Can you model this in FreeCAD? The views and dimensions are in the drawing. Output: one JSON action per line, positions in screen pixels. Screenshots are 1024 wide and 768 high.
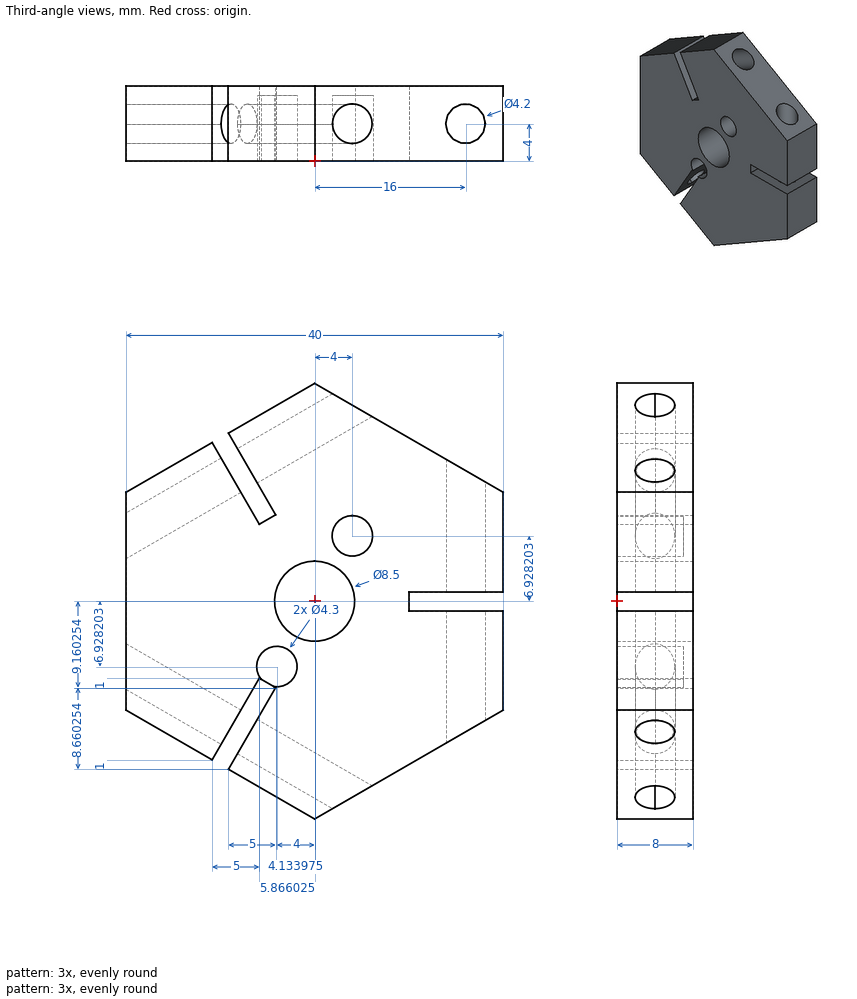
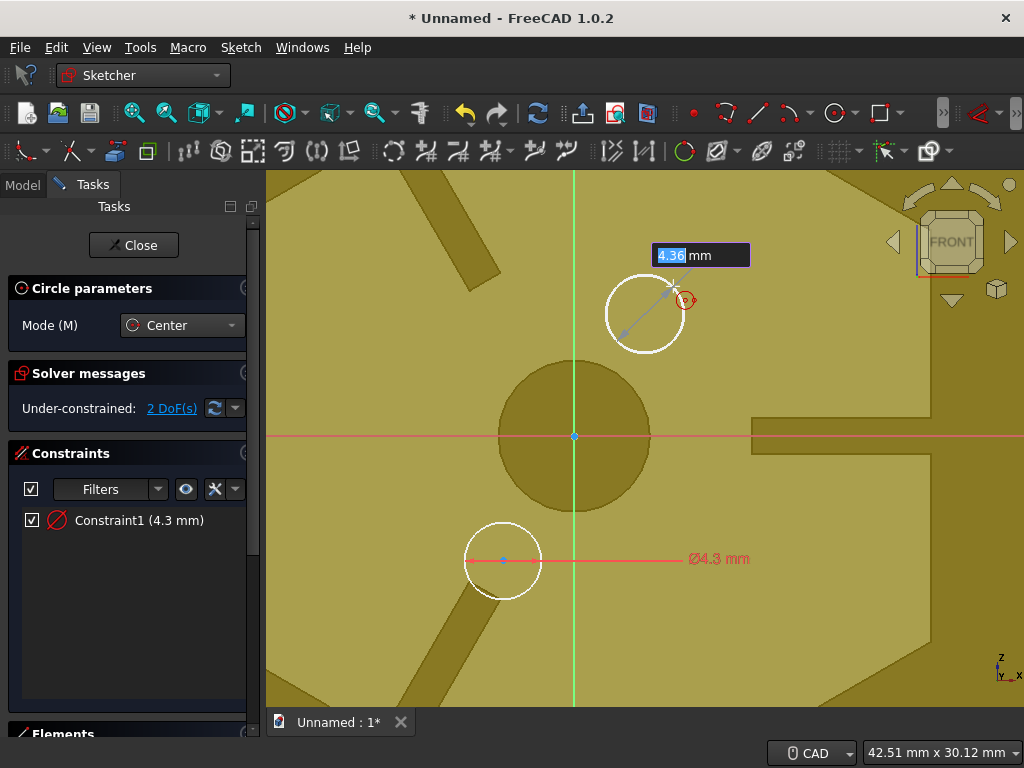
{"action": "type", "text": "4.3"}
{"action": "key", "text": "Return"}
{"action": "key", "text": "Escape"}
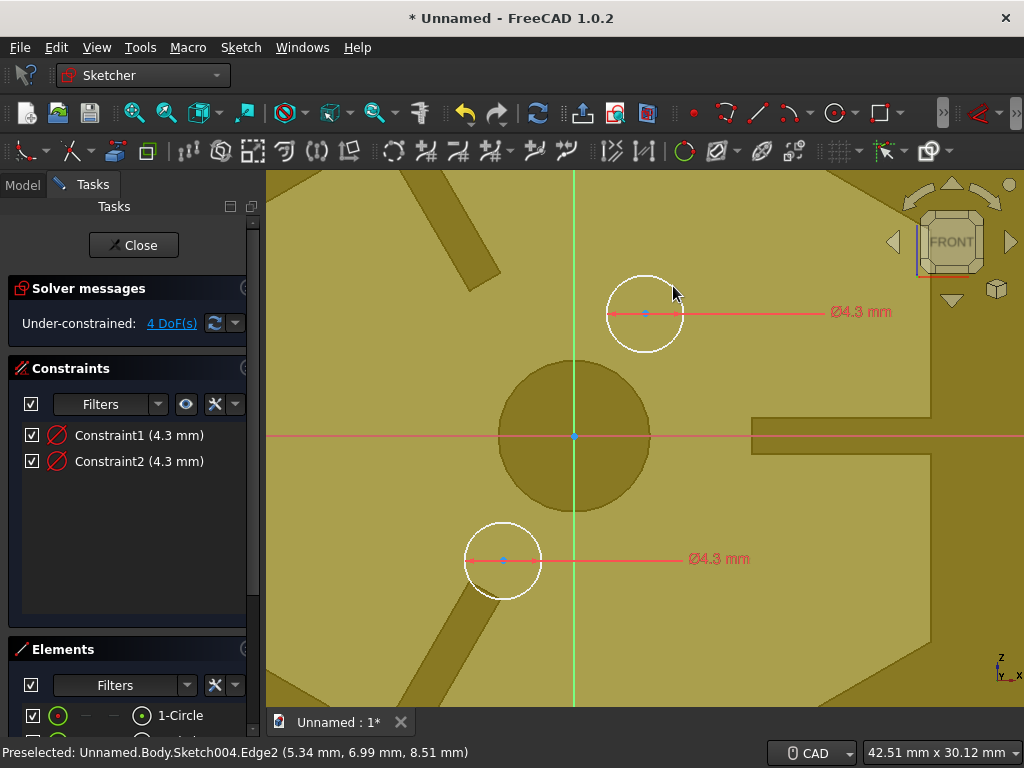
{"action": "left_click", "coordinate": [978, 114]}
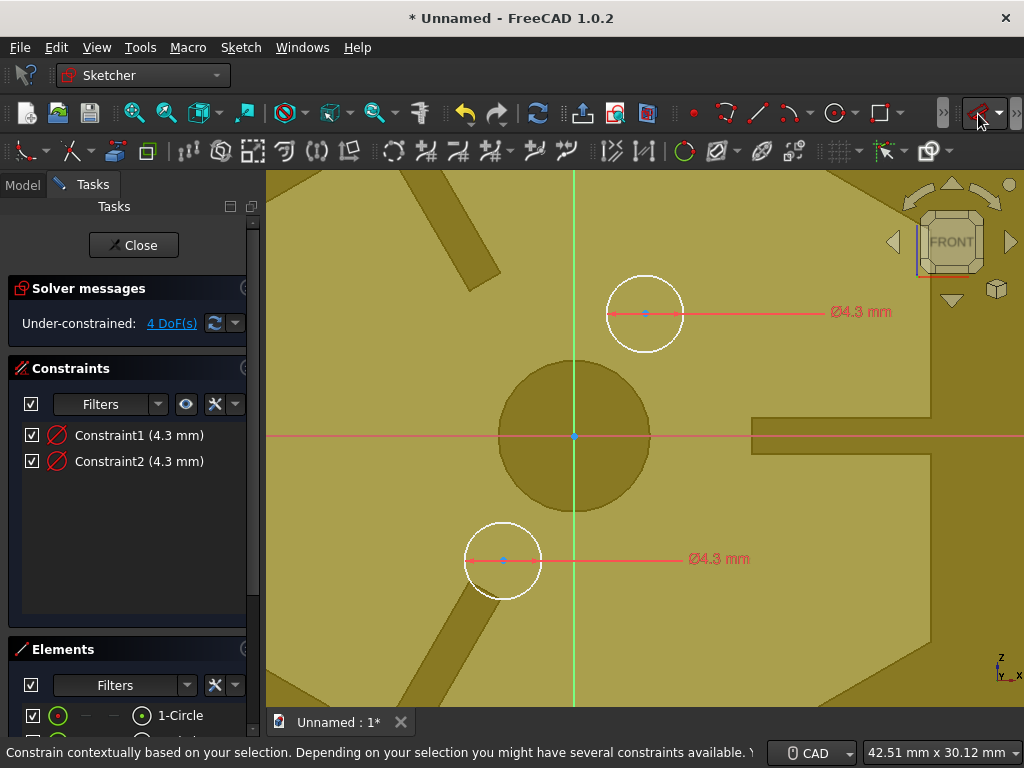
{"action": "left_click", "coordinate": [503, 561]}
{"action": "left_click", "coordinate": [555, 595]}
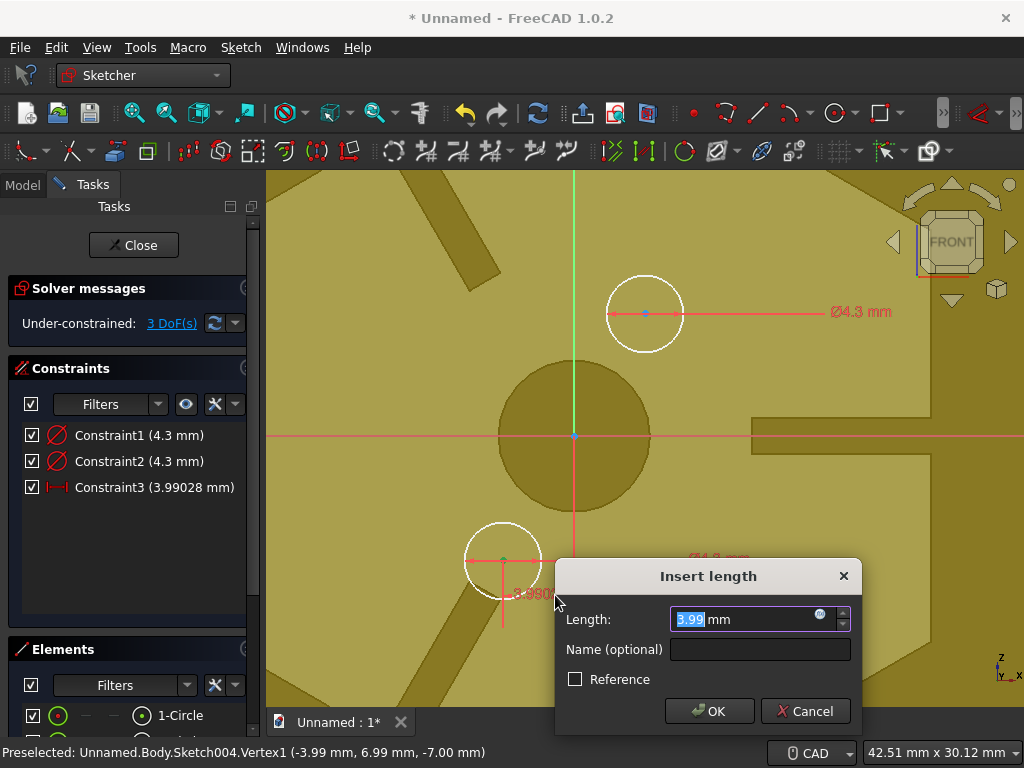
{"action": "type", "text": "4"}
{"action": "key", "text": "Return"}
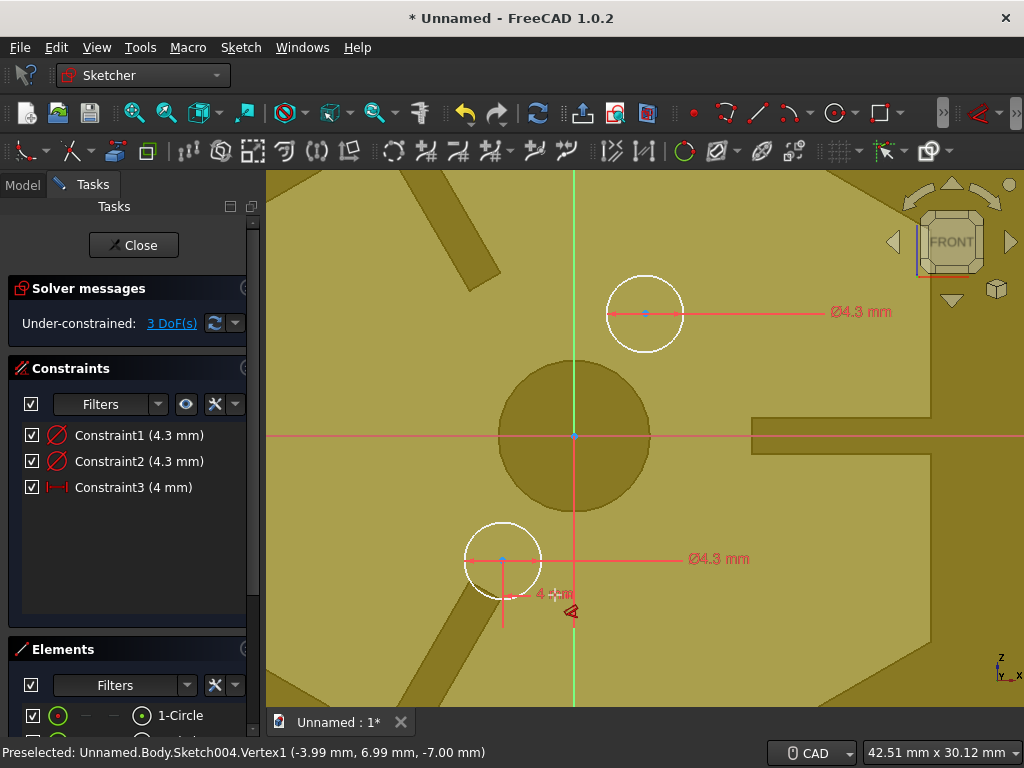
{"action": "left_click", "coordinate": [645, 314]}
{"action": "left_click", "coordinate": [593, 280]}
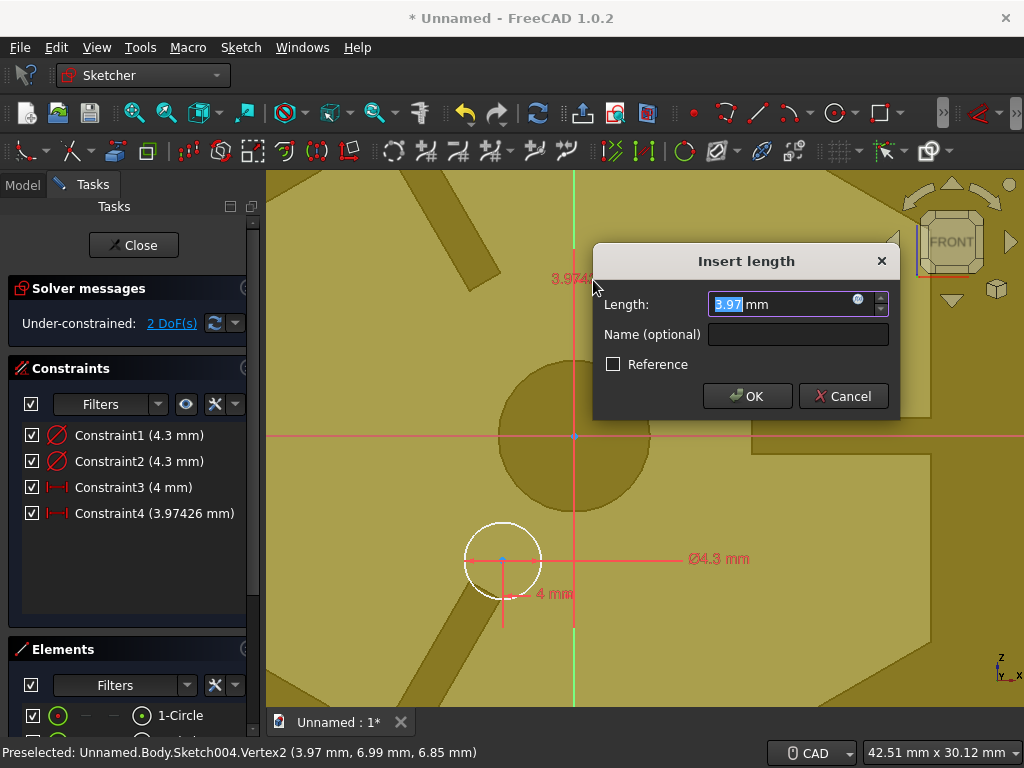
{"action": "type", "text": "4"}
{"action": "key", "text": "Return"}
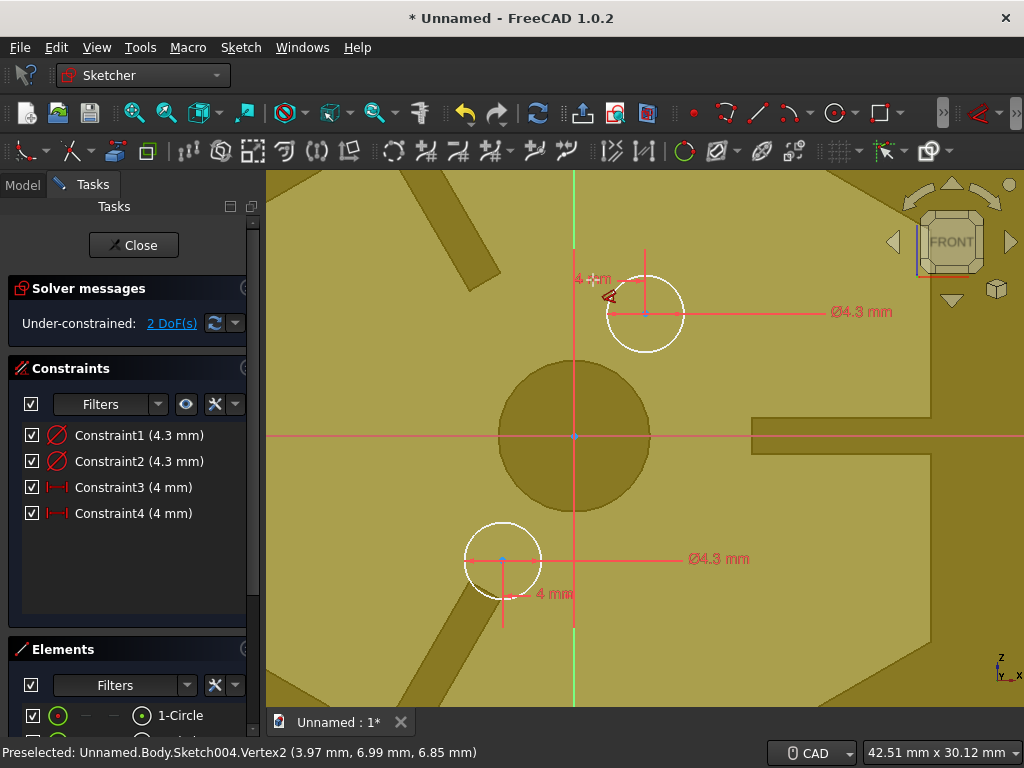
{"action": "left_click", "coordinate": [503, 561]}
{"action": "left_click", "coordinate": [469, 499]}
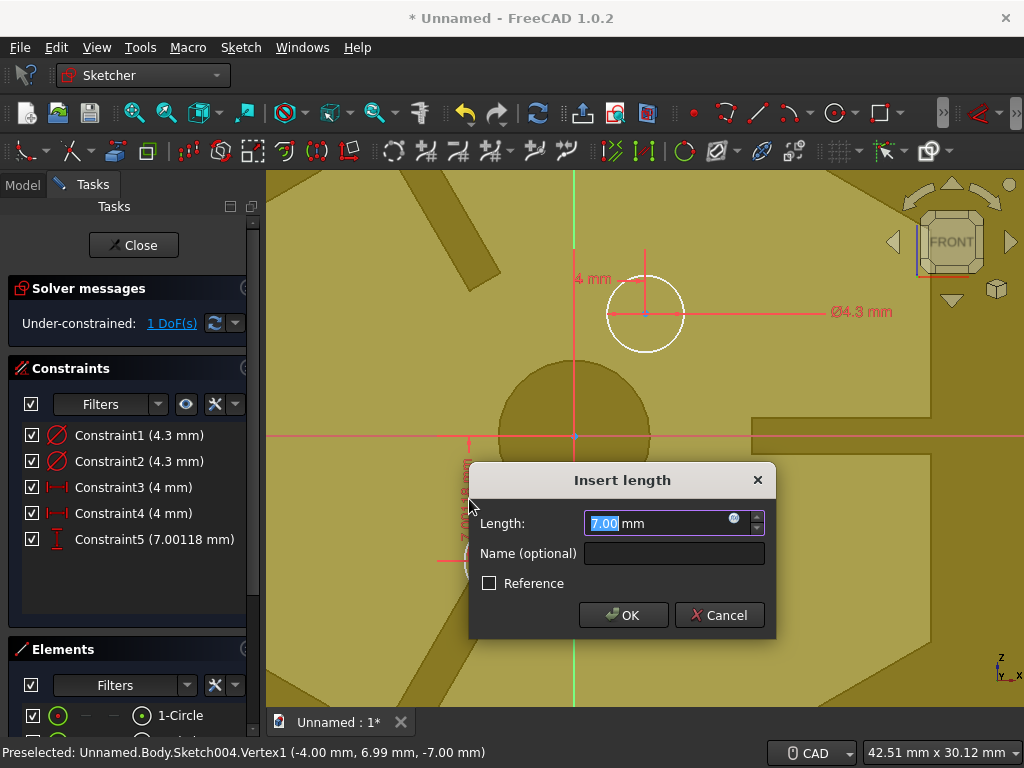
{"action": "type", "text": "6.928203"}
{"action": "key", "text": "Return"}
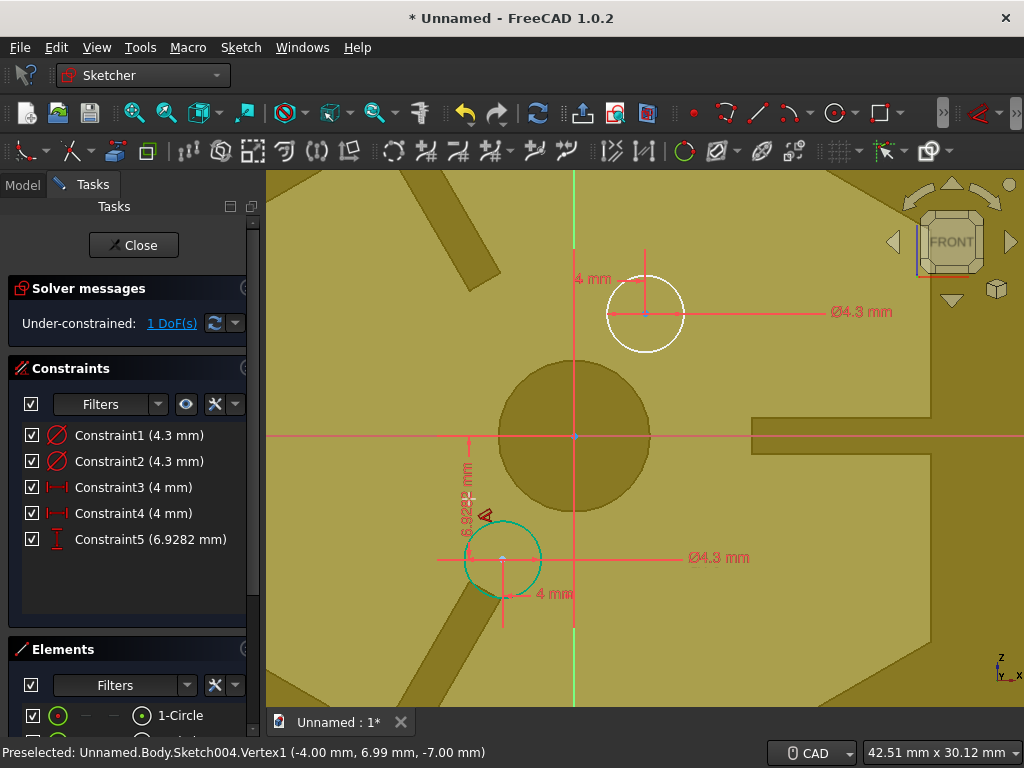
{"action": "left_click", "coordinate": [645, 314]}
{"action": "left_click", "coordinate": [679, 375]}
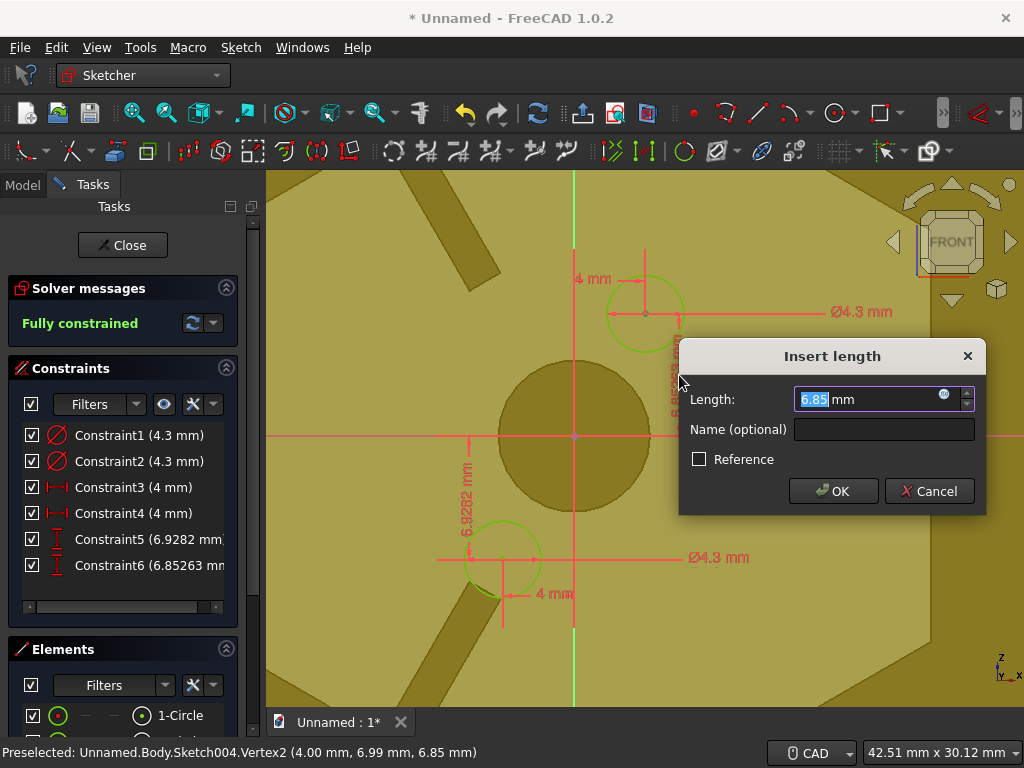
{"action": "type", "text": "6.928203"}
{"action": "key", "text": "Return"}
{"action": "key", "text": "Escape"}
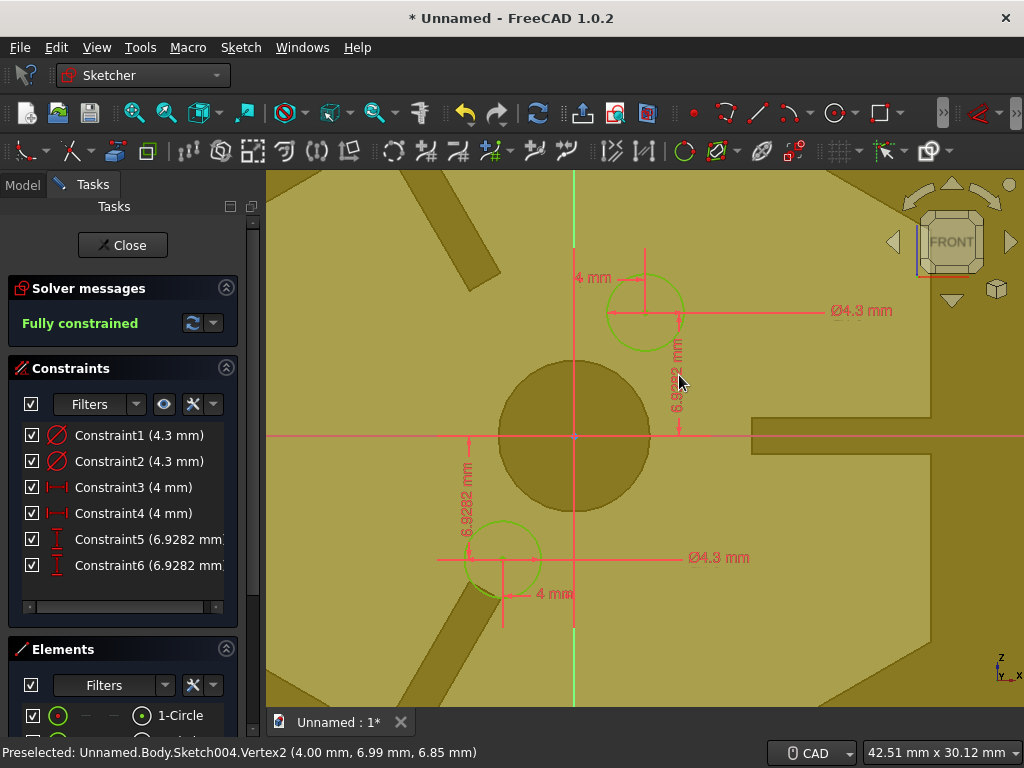
{"action": "left_click", "coordinate": [123, 245]}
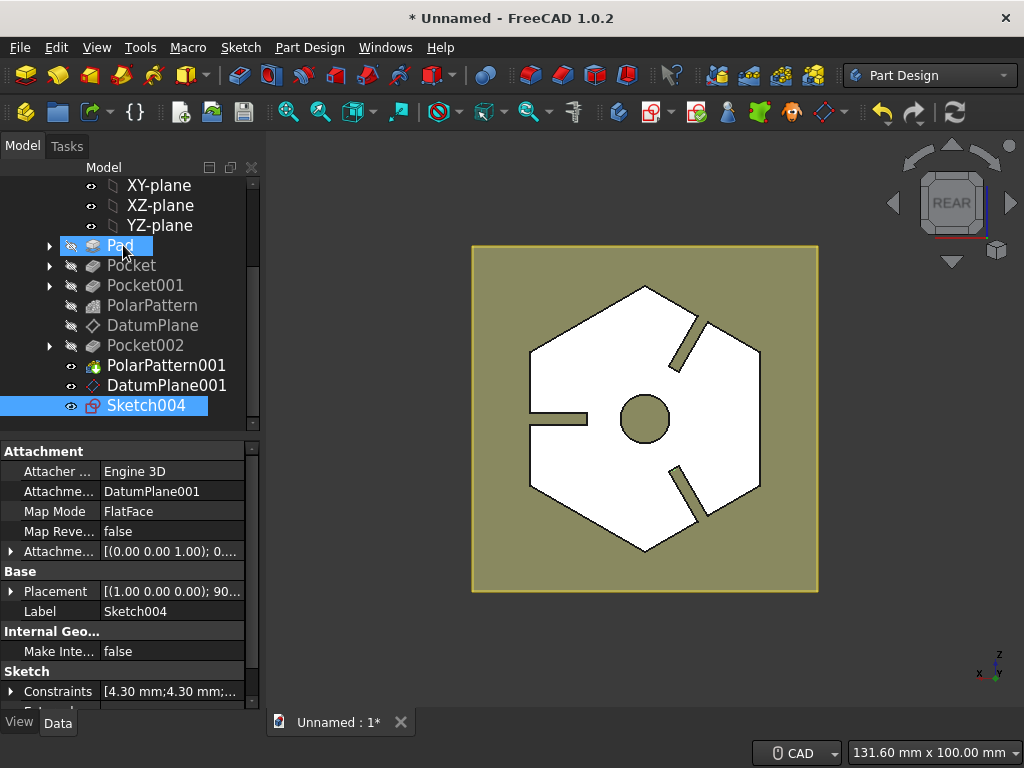
{"action": "left_click", "coordinate": [240, 76]}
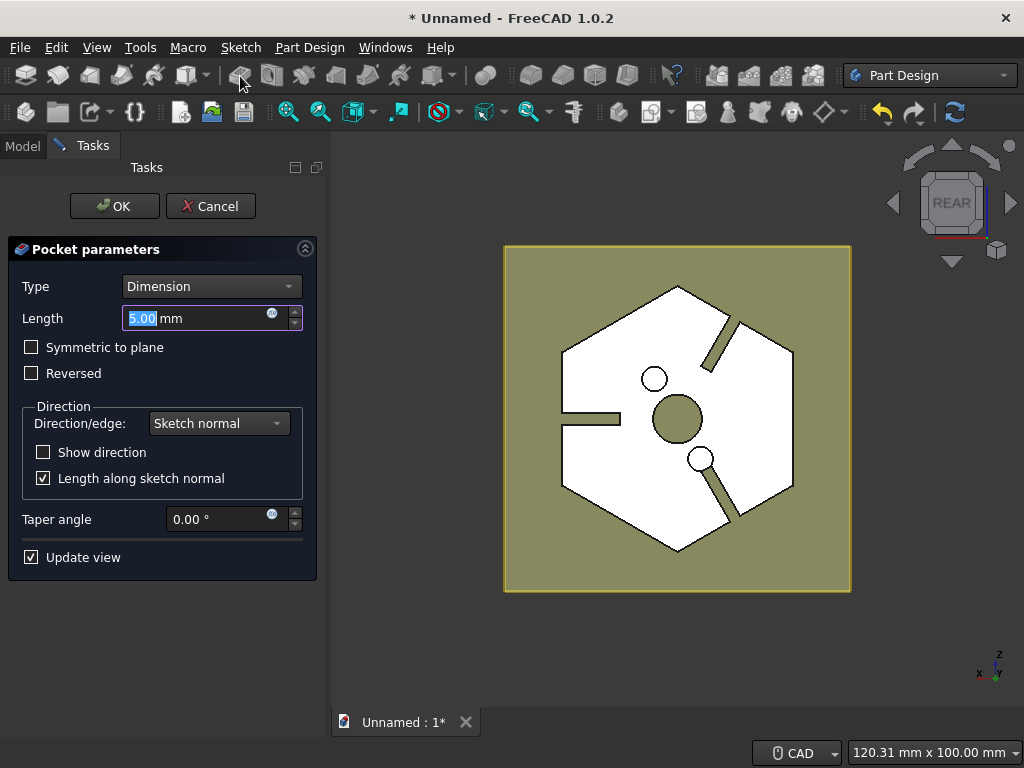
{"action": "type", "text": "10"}
{"action": "key", "text": "Tab"}